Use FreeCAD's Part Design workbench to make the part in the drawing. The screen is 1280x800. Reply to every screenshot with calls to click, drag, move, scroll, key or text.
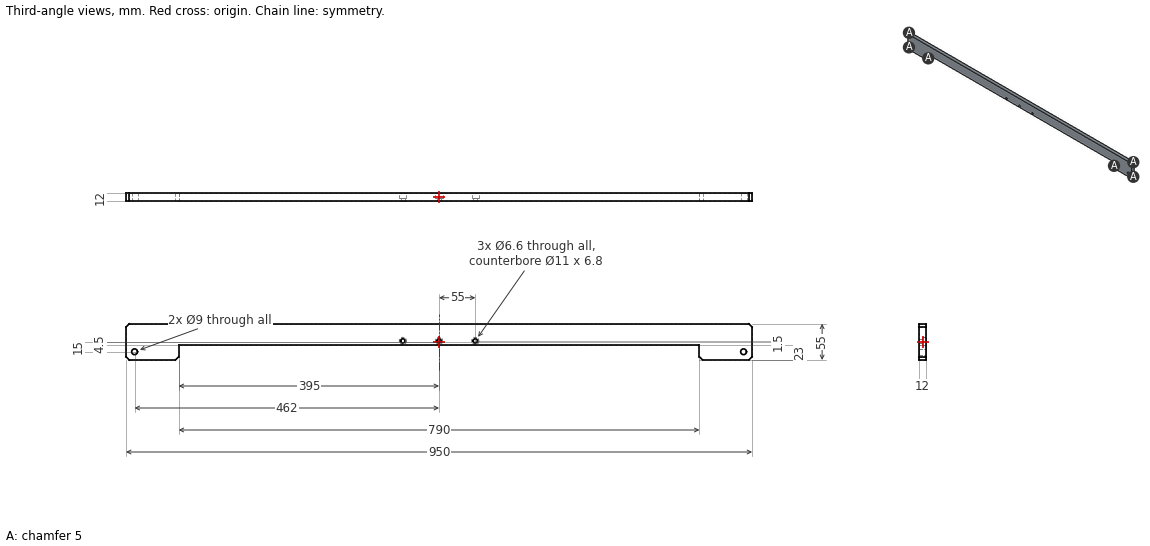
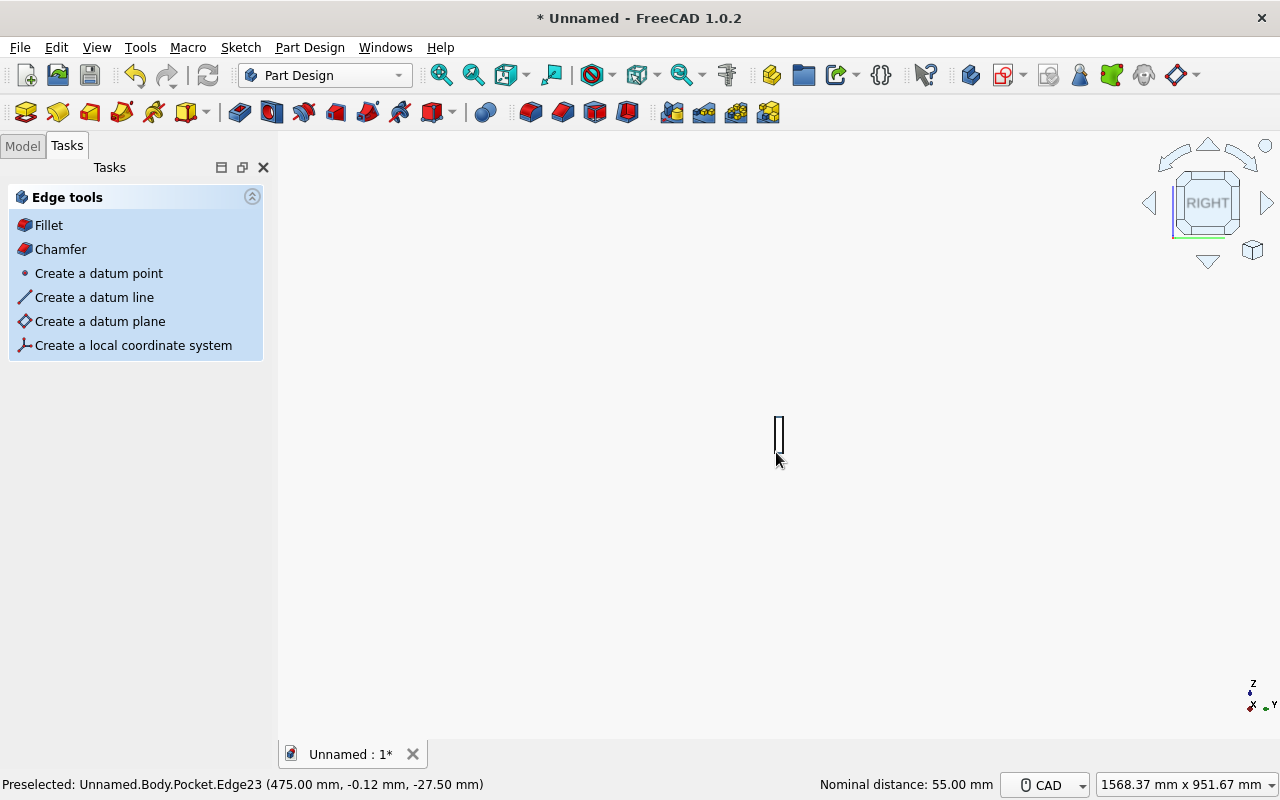
key(5)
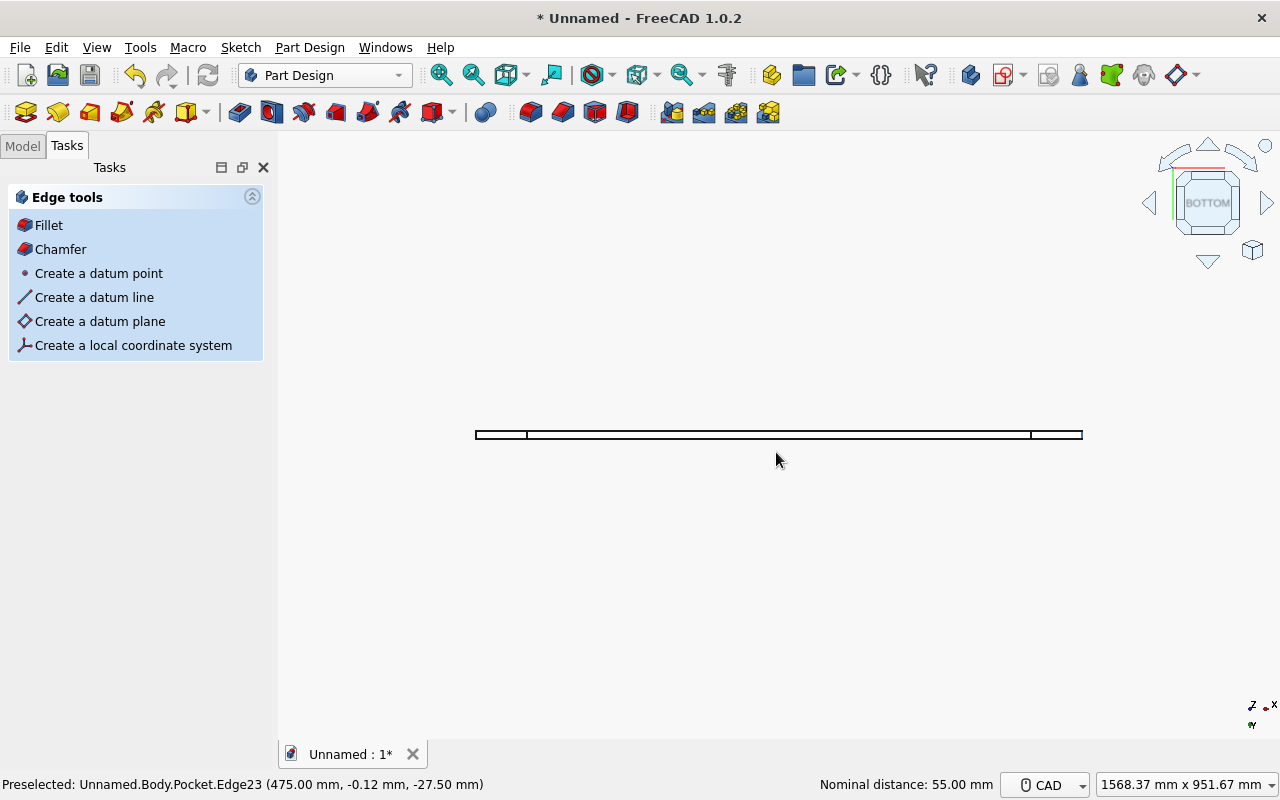
scroll(527, 434, up, 9)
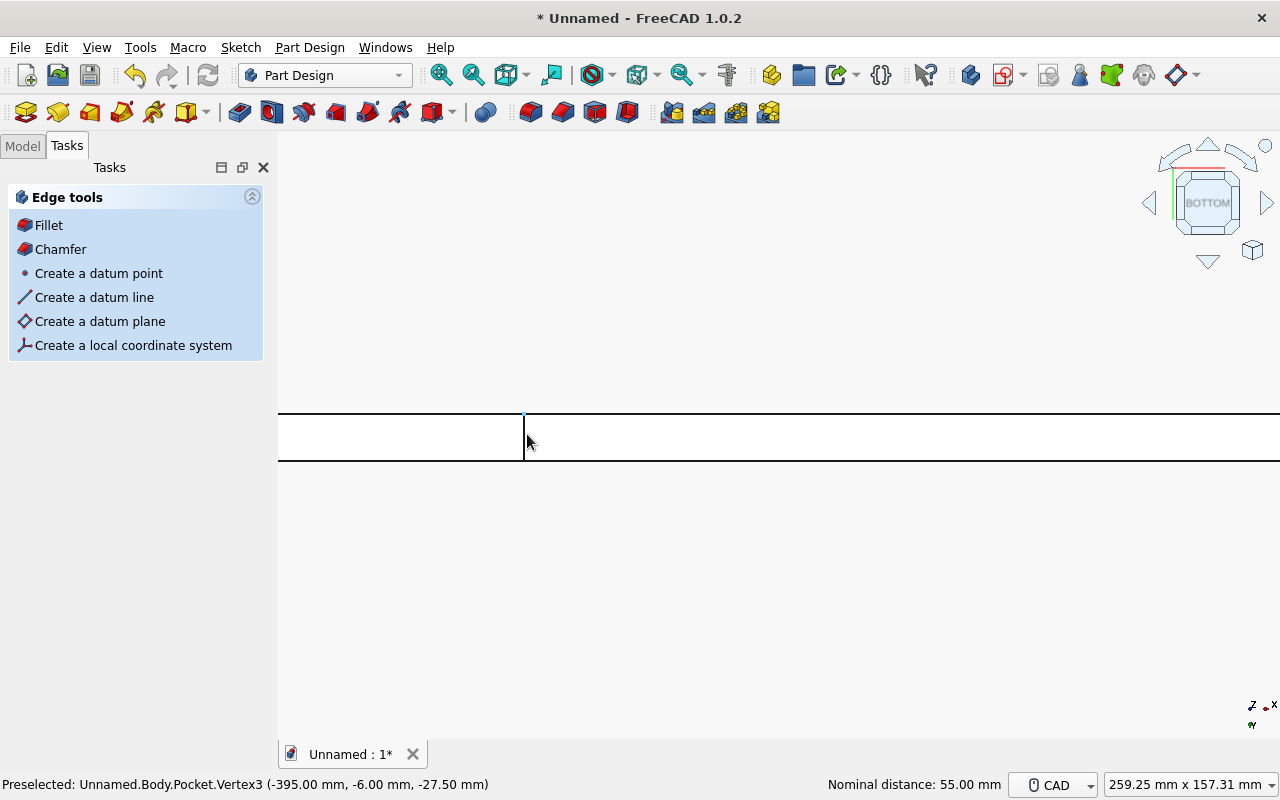
click(524, 437, ctrl)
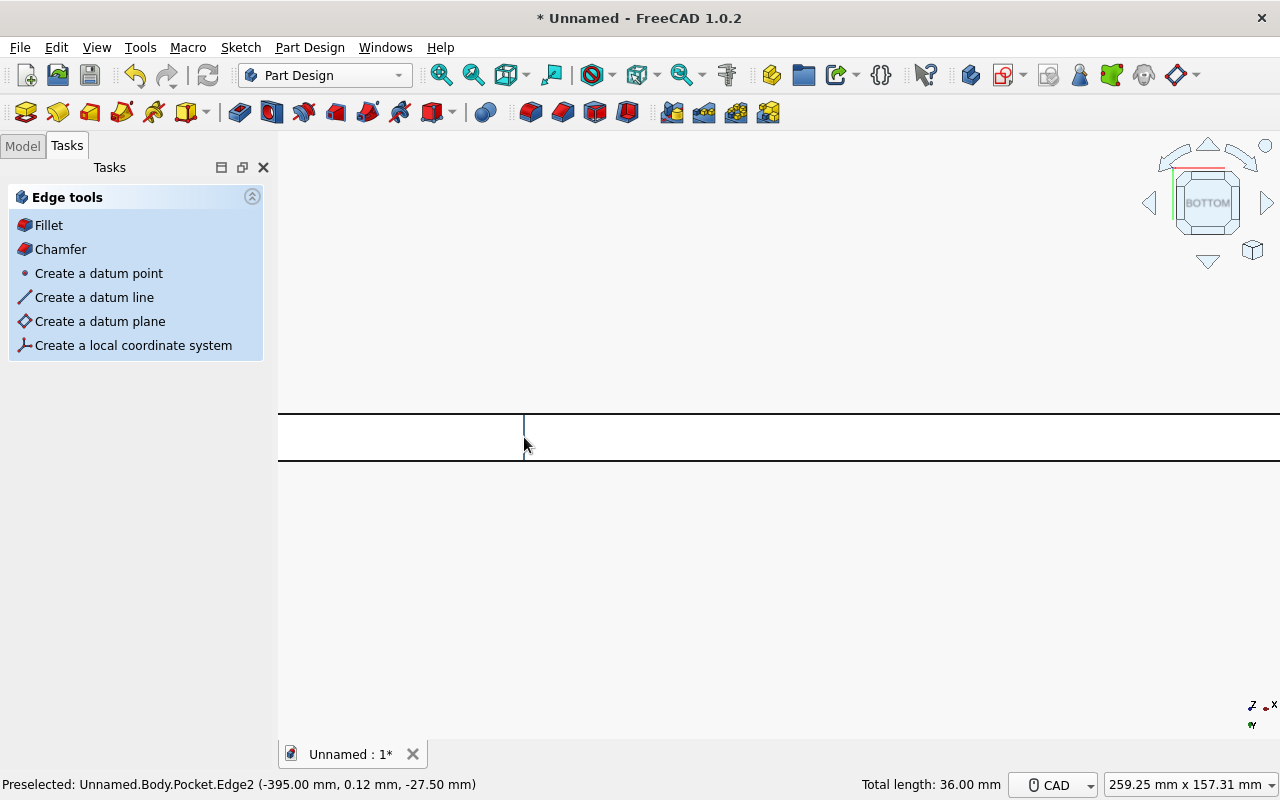
key(v)
key(f)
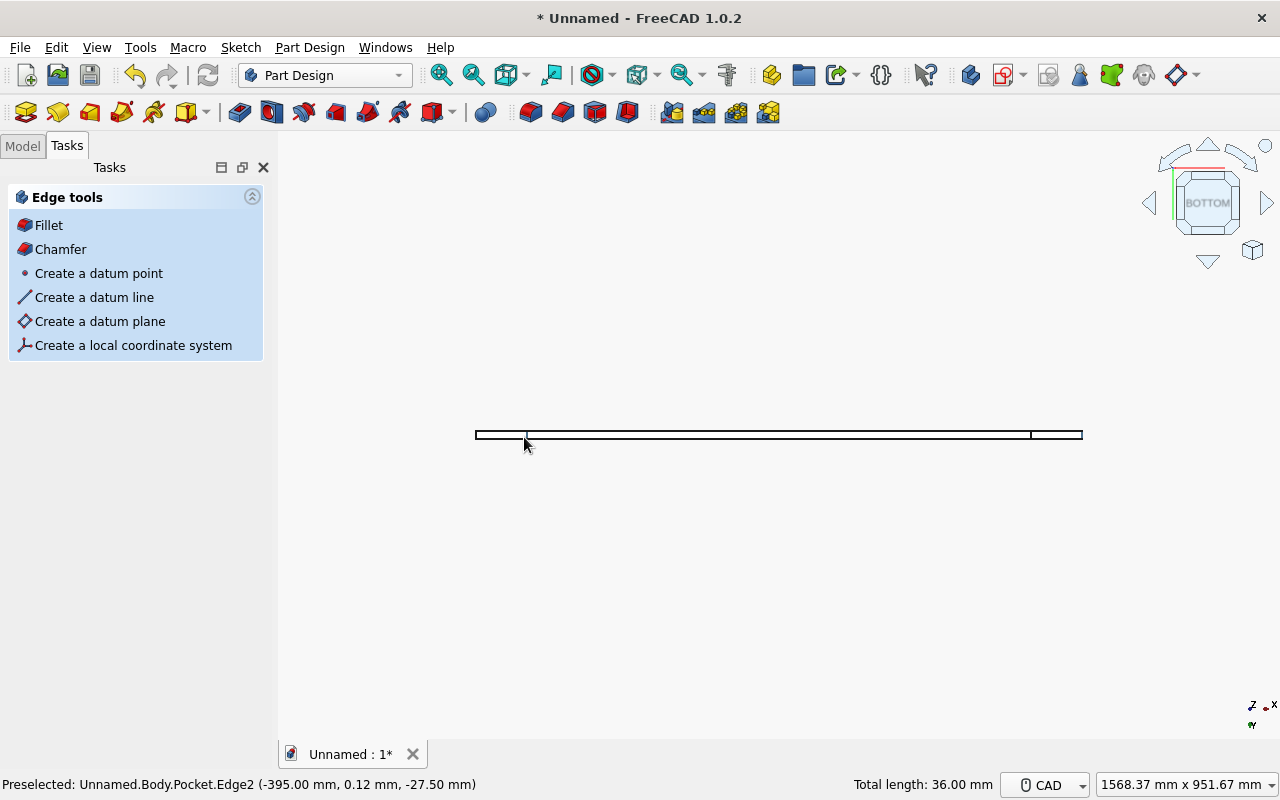
key(4)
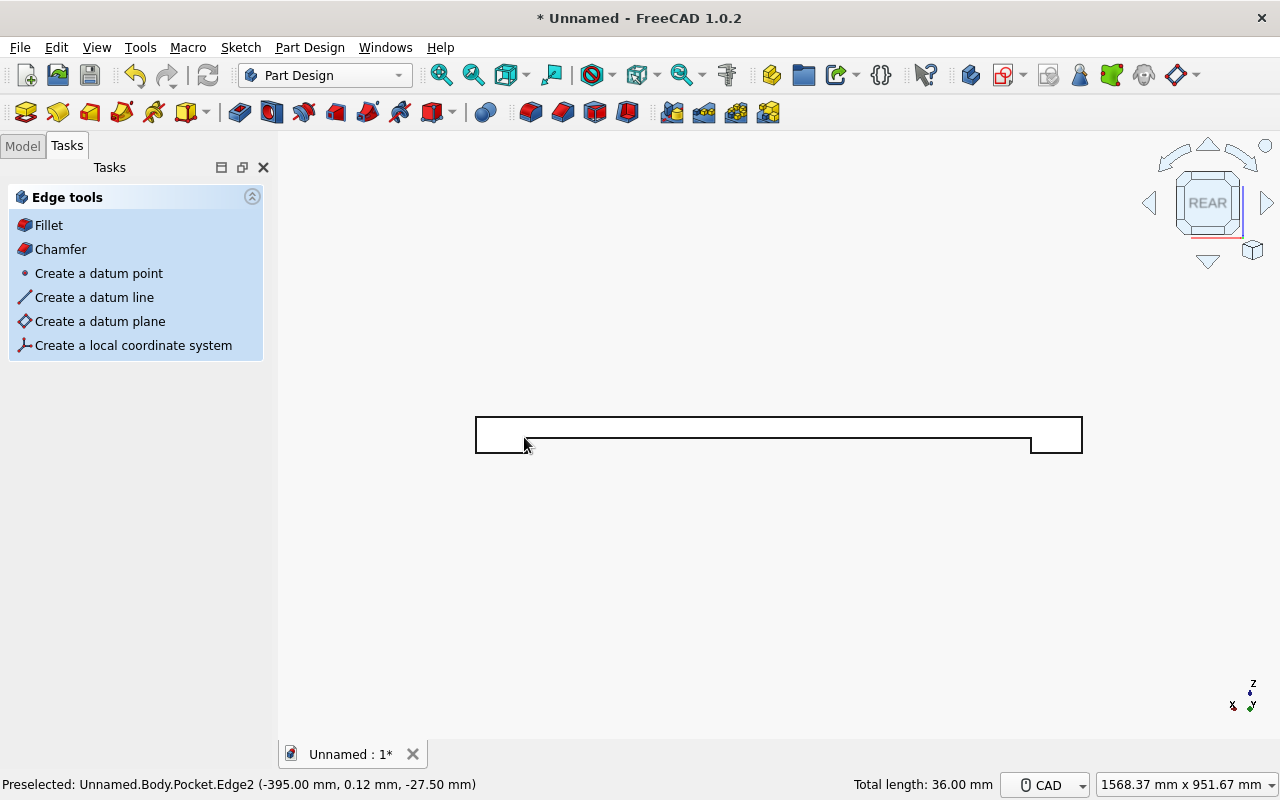
scroll(527, 452, up, 9)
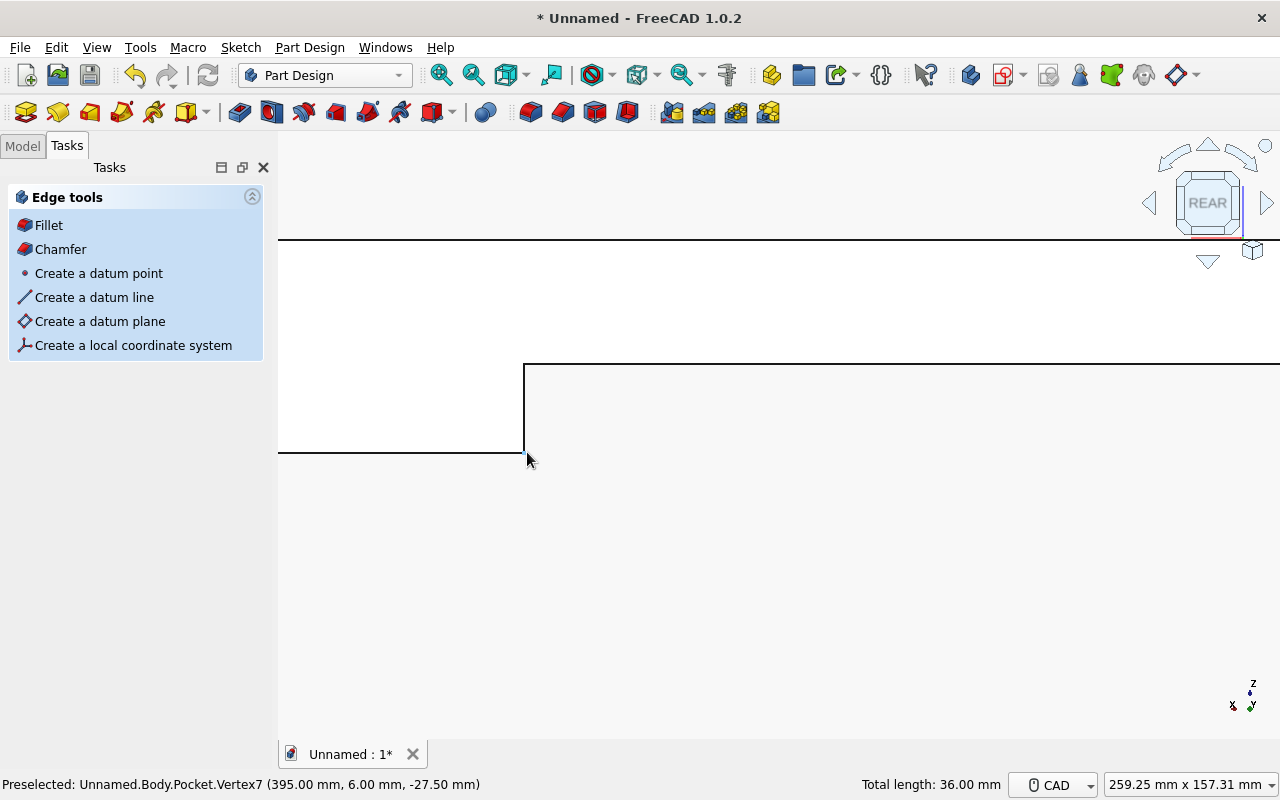
key(v)
key(f)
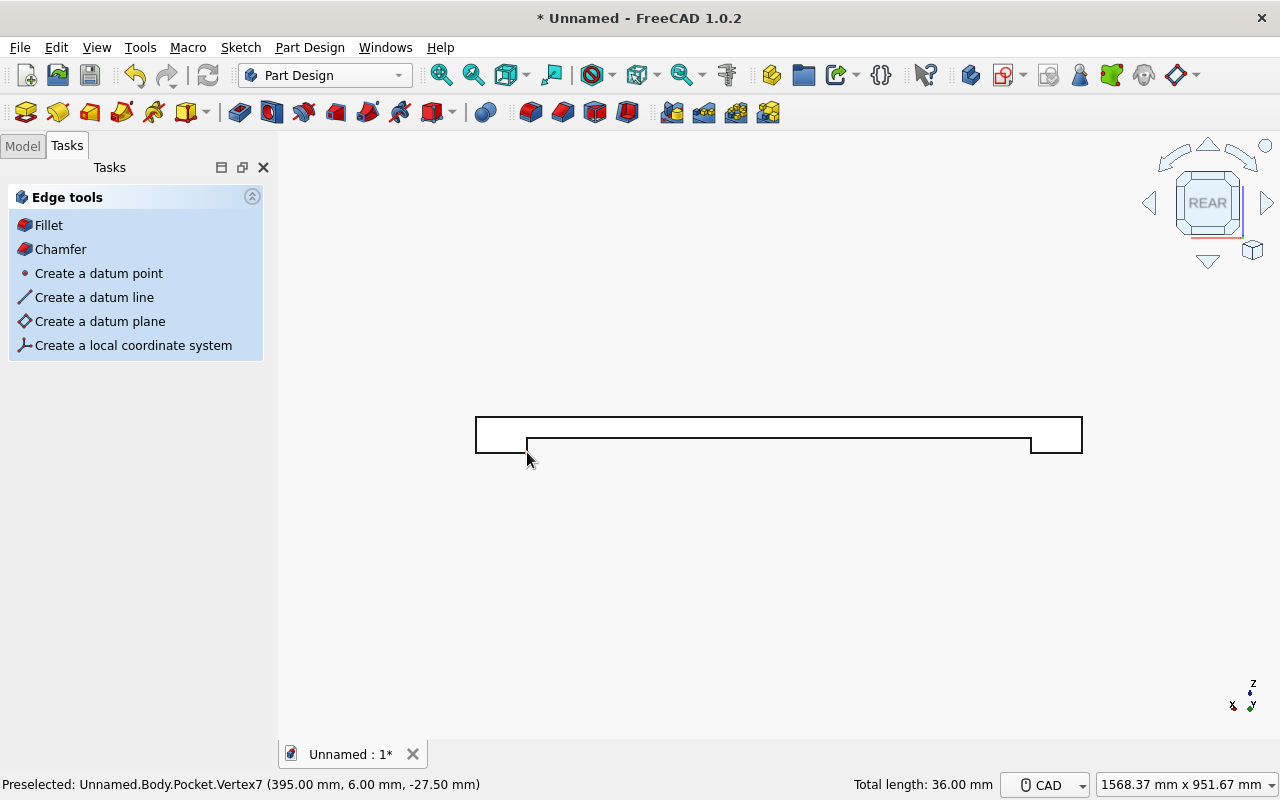
key(6)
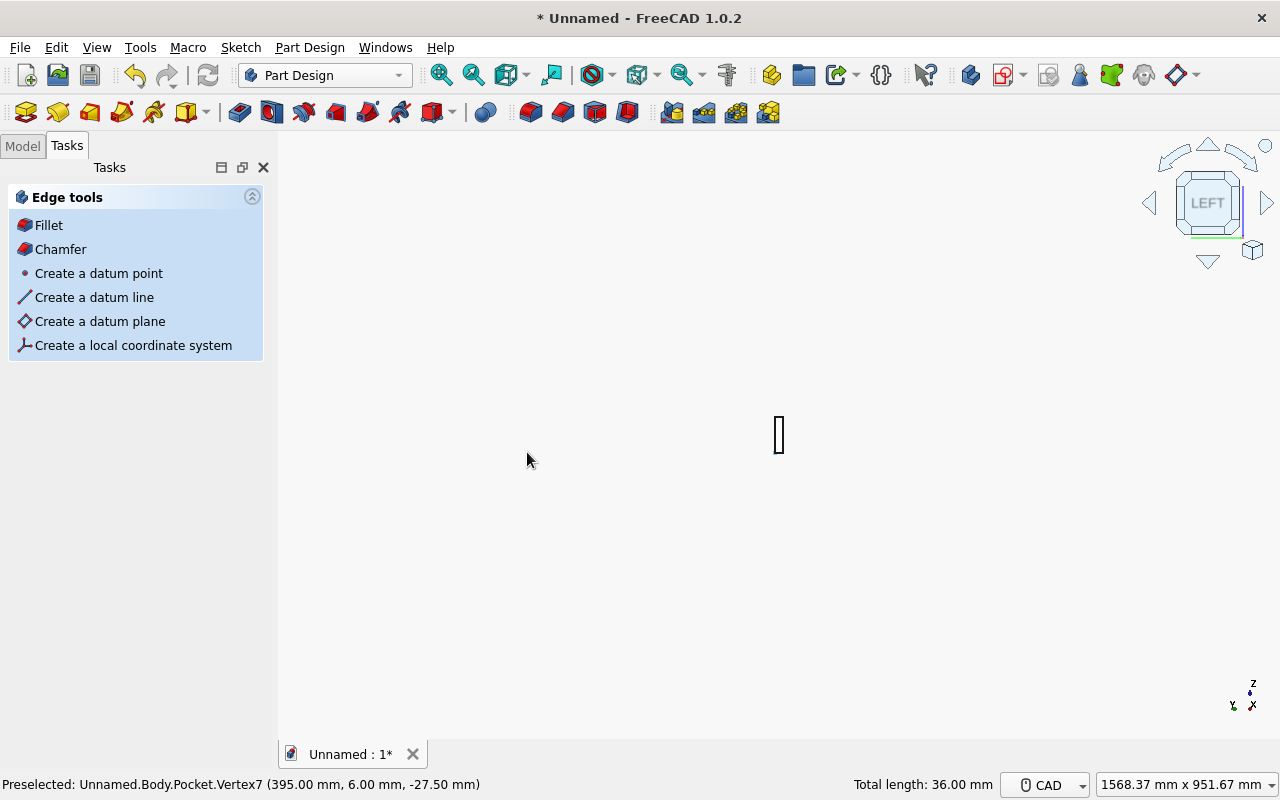
key(v)
key(f)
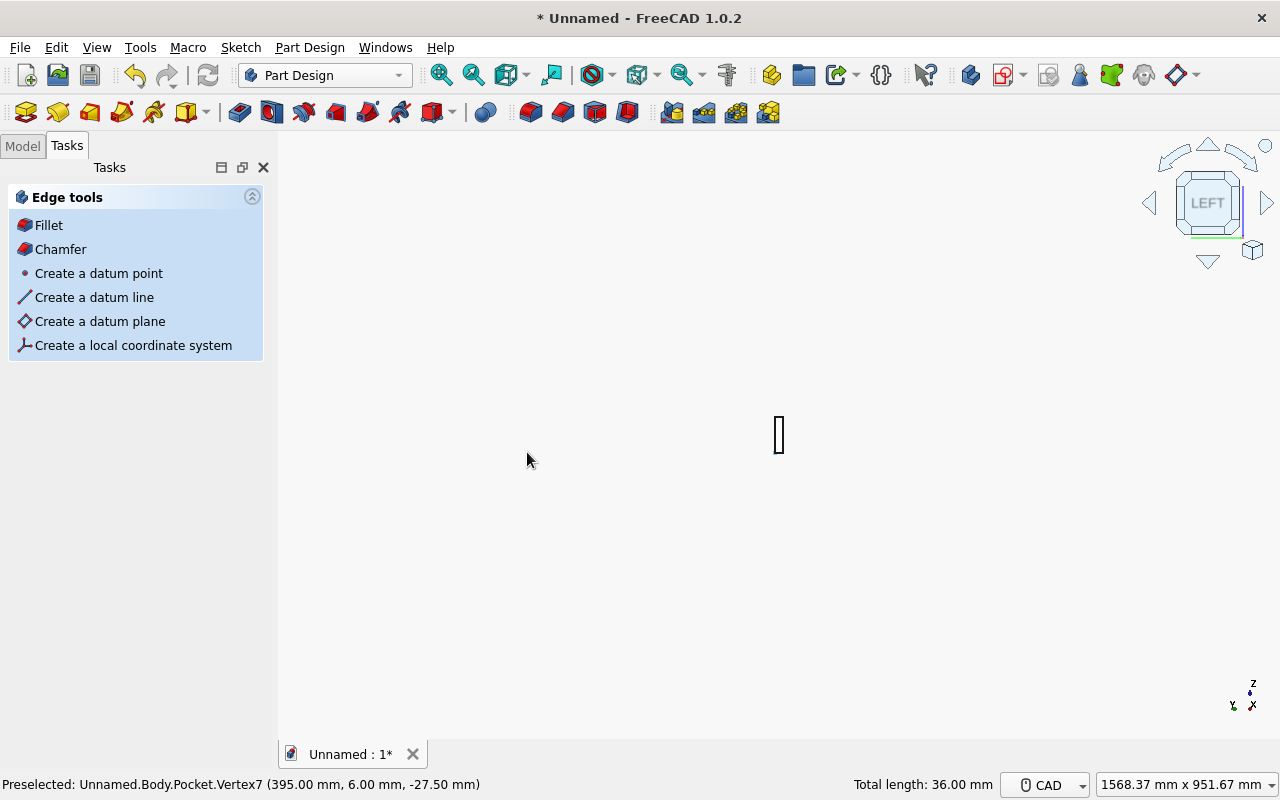
scroll(779, 452, up, 9)